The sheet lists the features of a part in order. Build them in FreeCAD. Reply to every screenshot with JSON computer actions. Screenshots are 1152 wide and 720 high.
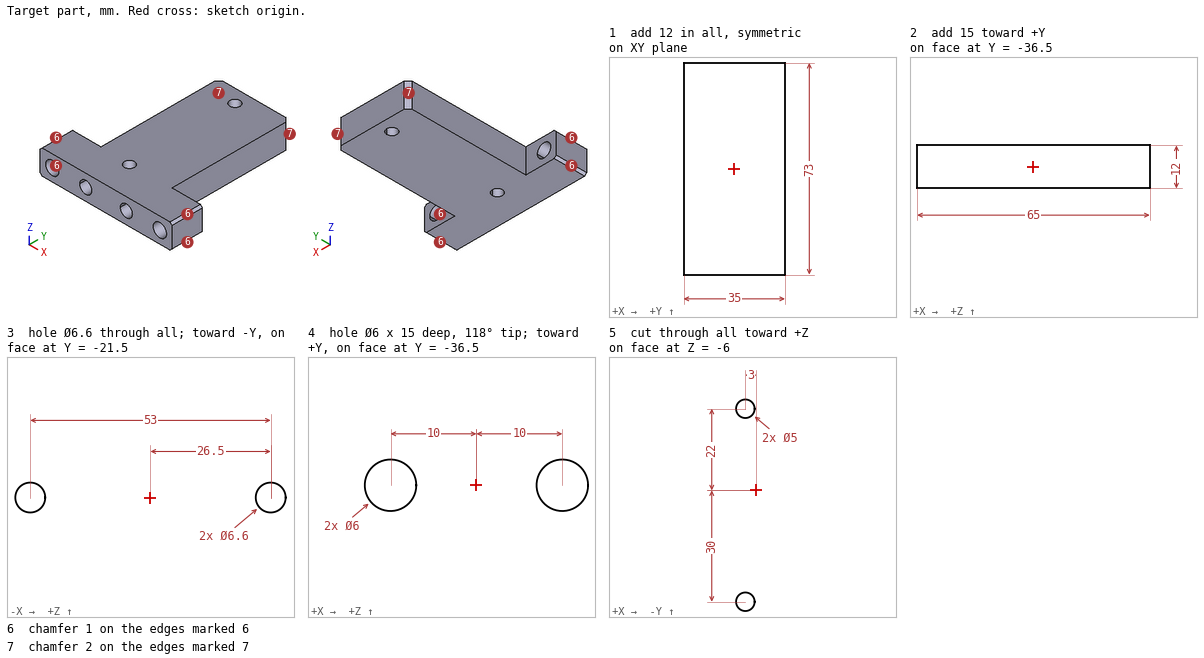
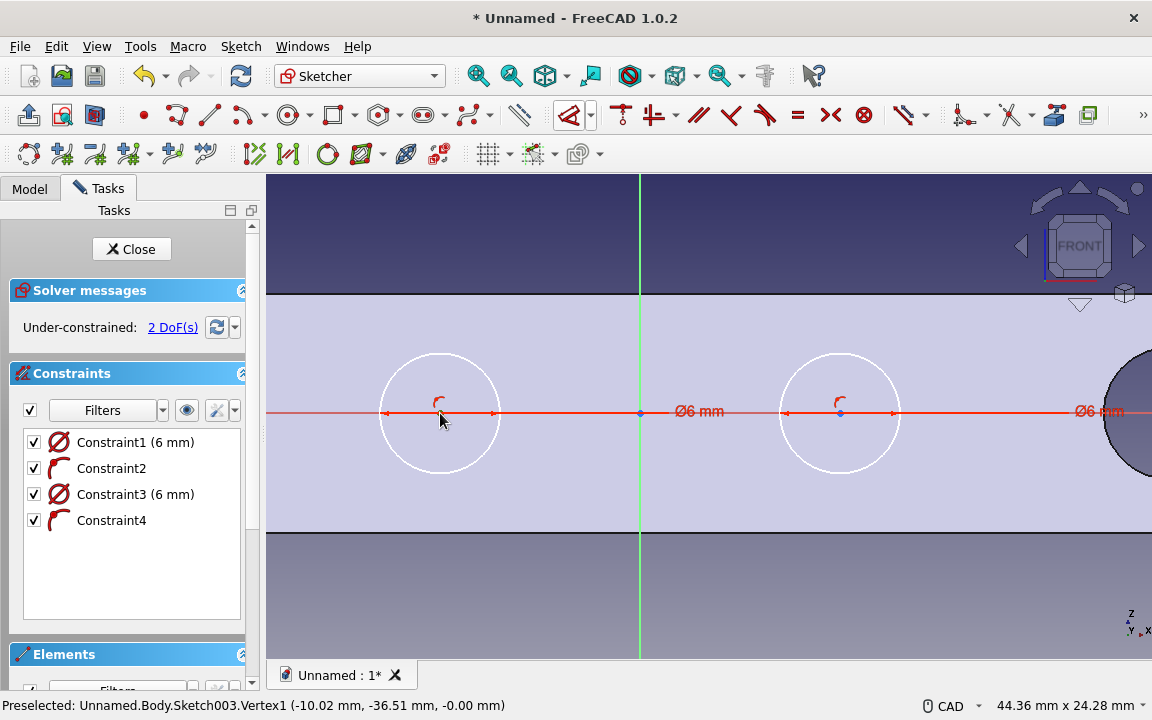
{"action": "key", "text": "l"}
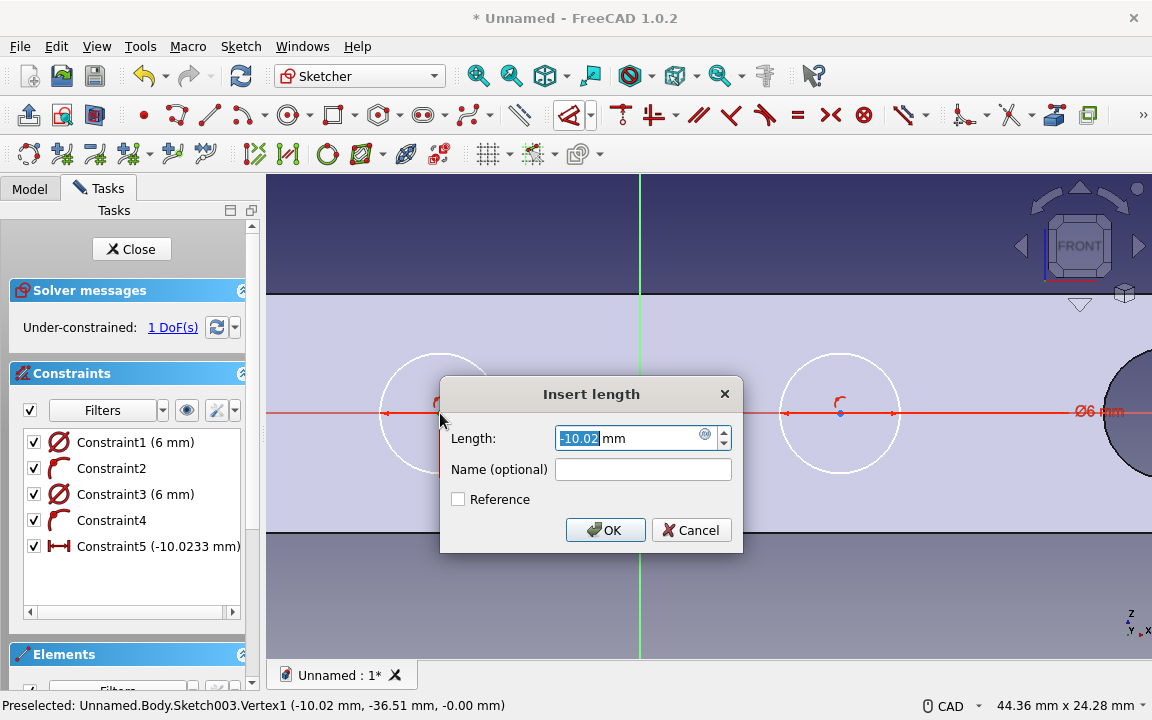
{"action": "type", "text": "-10"}
{"action": "key", "text": "Return"}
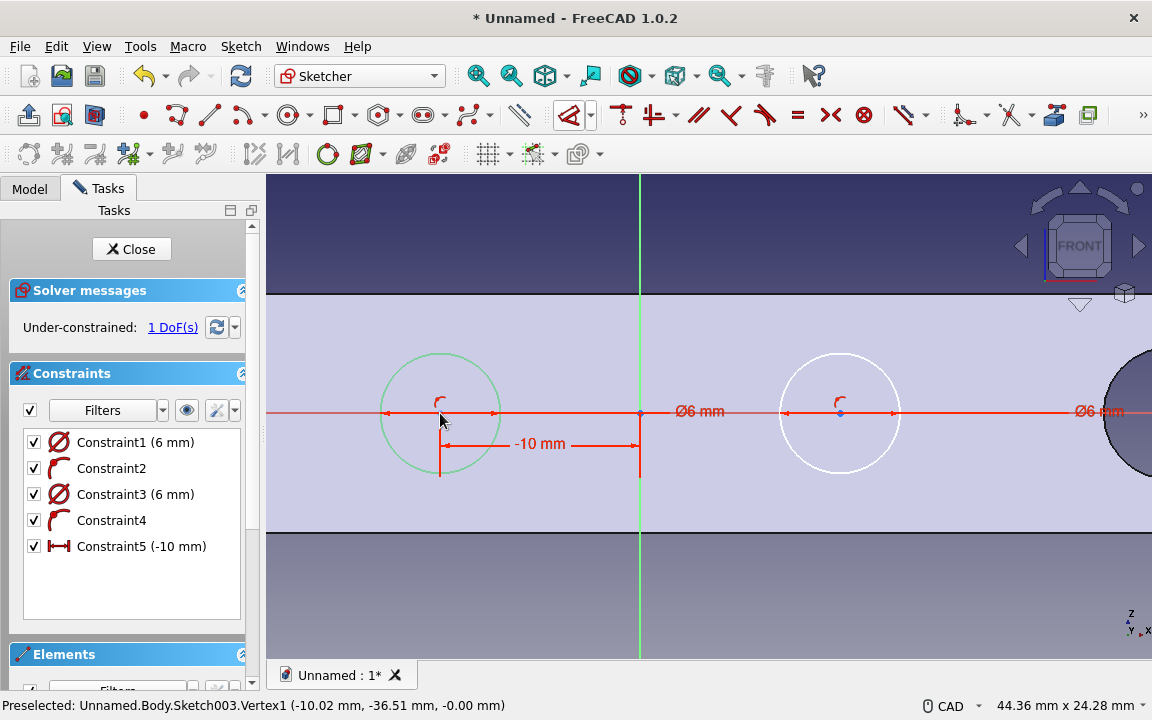
{"action": "left_click", "coordinate": [840, 413]}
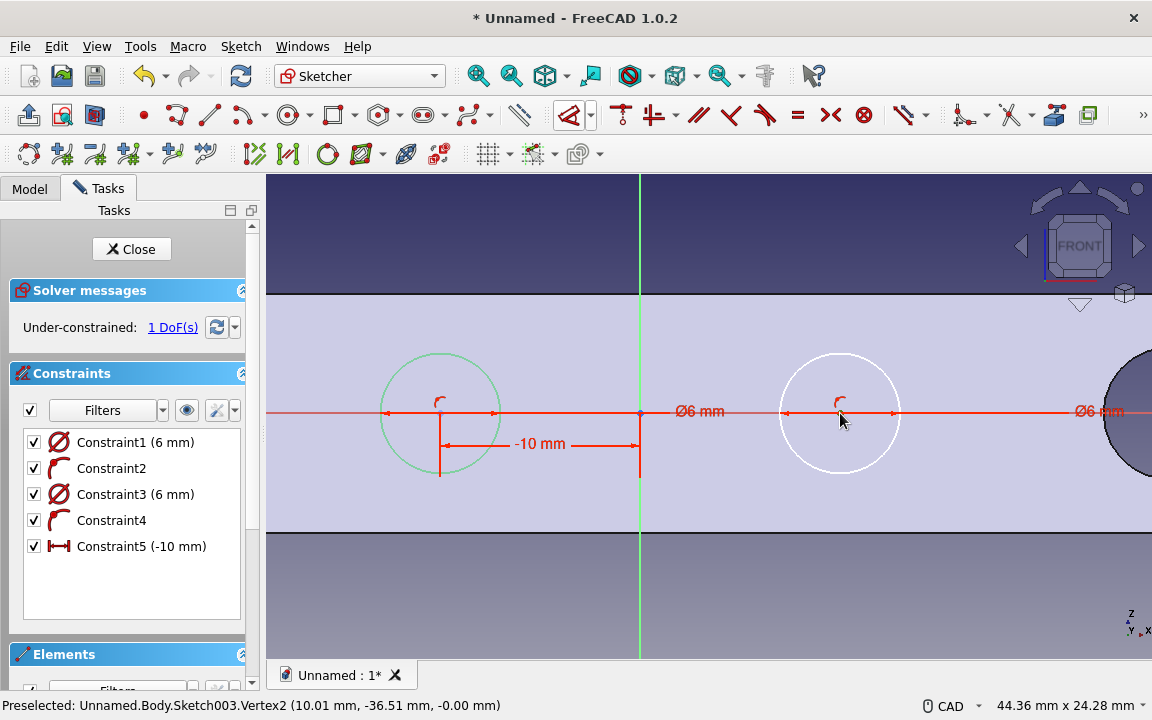
{"action": "left_click", "coordinate": [590, 116]}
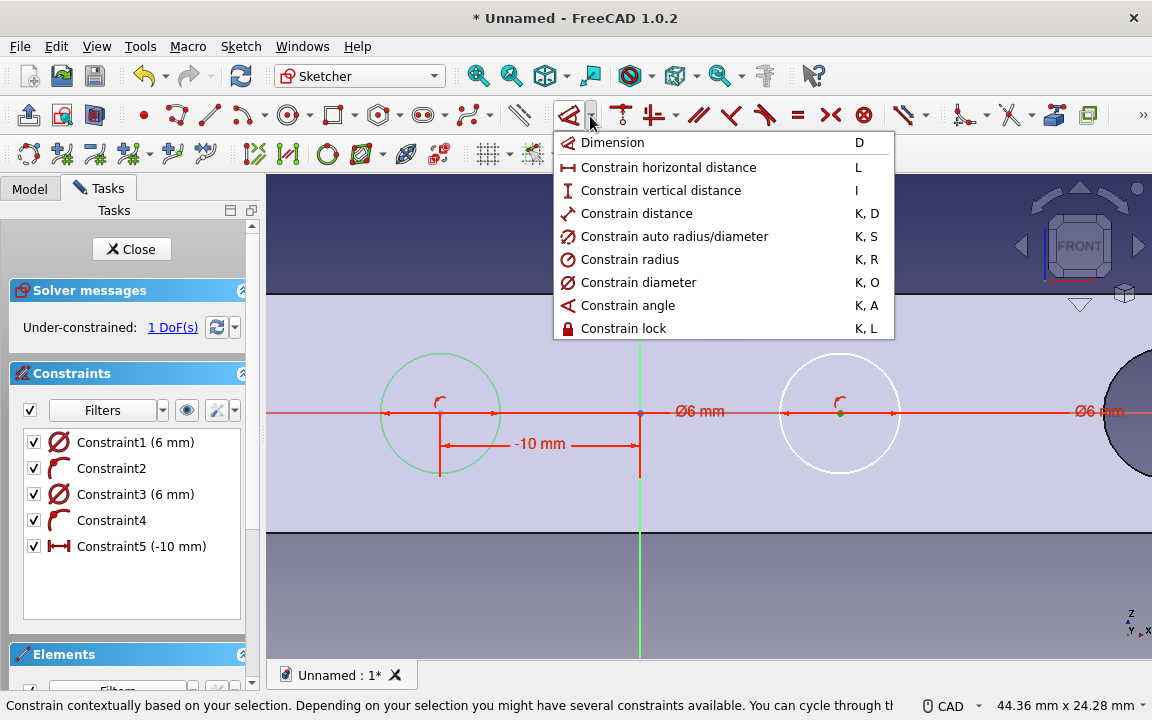
{"action": "left_click", "coordinate": [724, 168]}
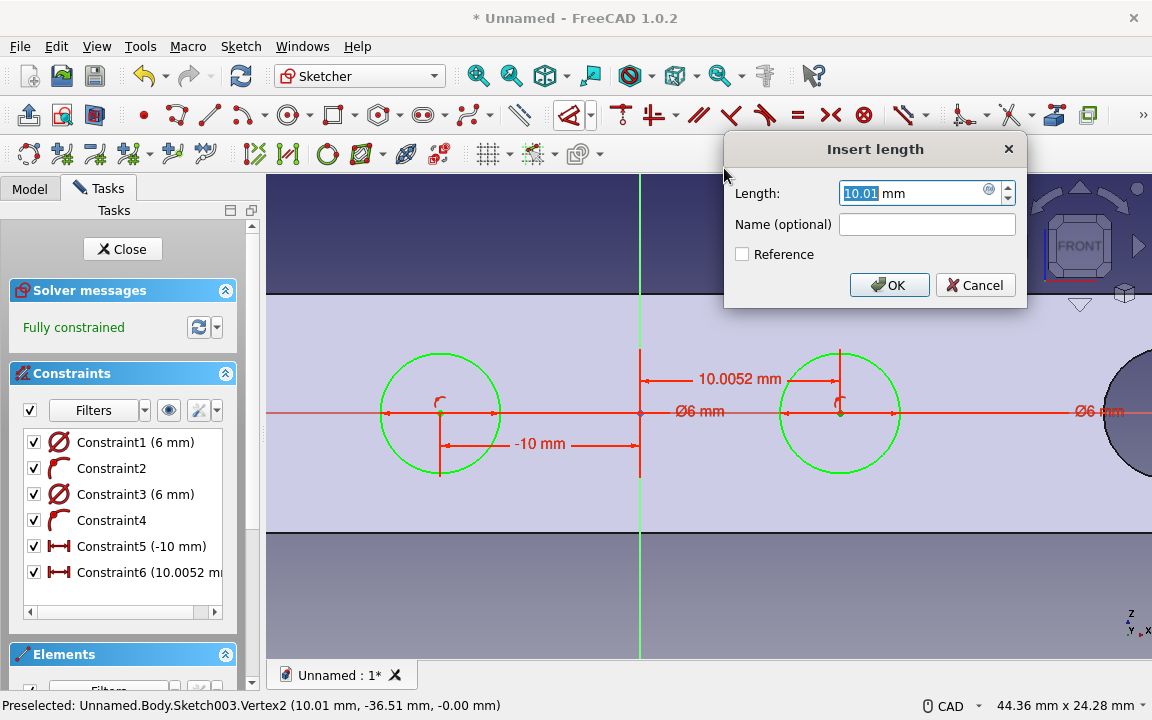
{"action": "type", "text": "10"}
{"action": "key", "text": "Return"}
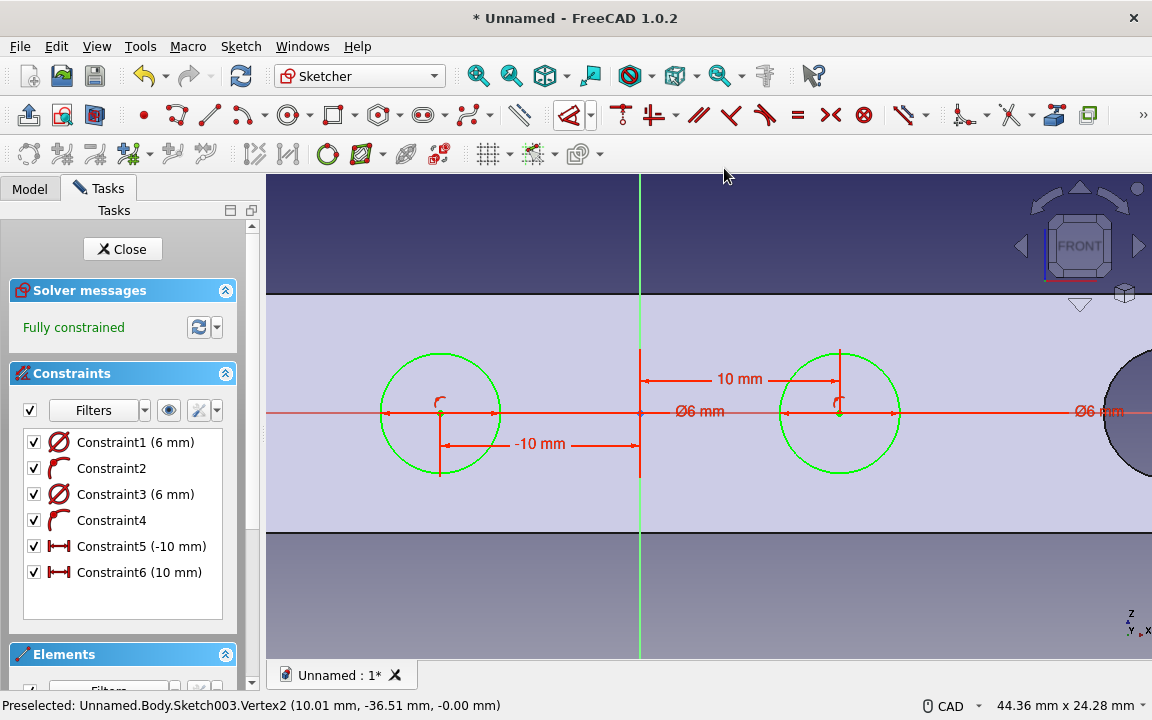
{"action": "left_click", "coordinate": [123, 249]}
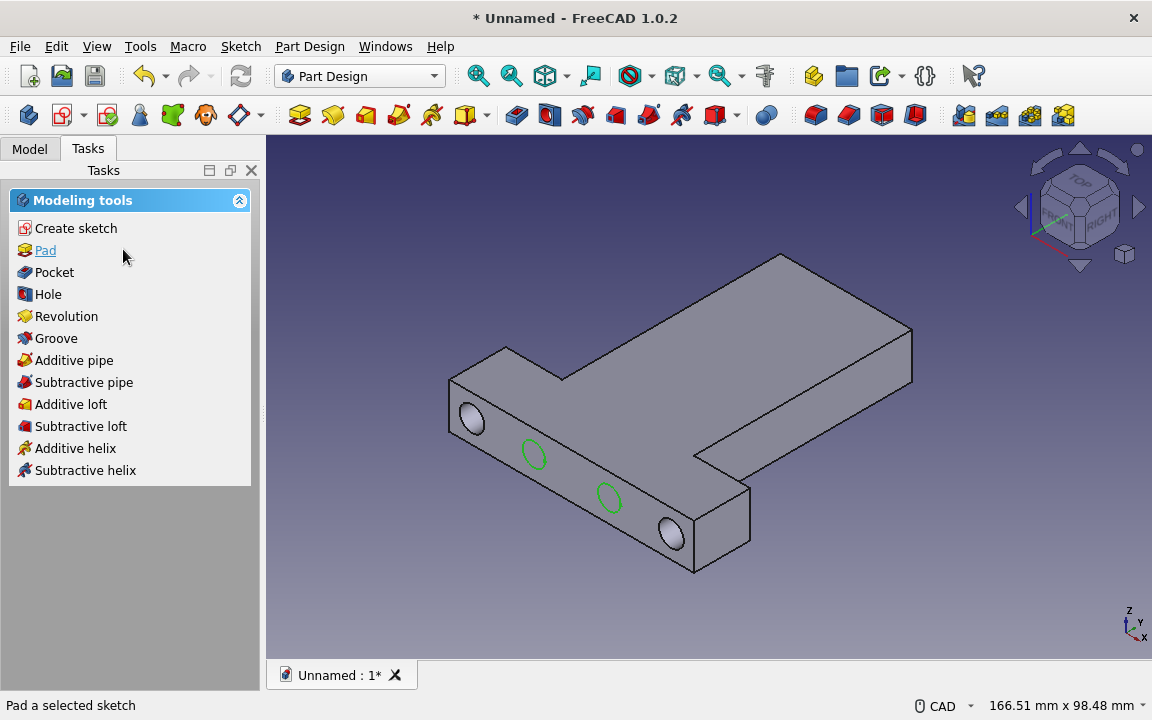
{"action": "left_click", "coordinate": [550, 116]}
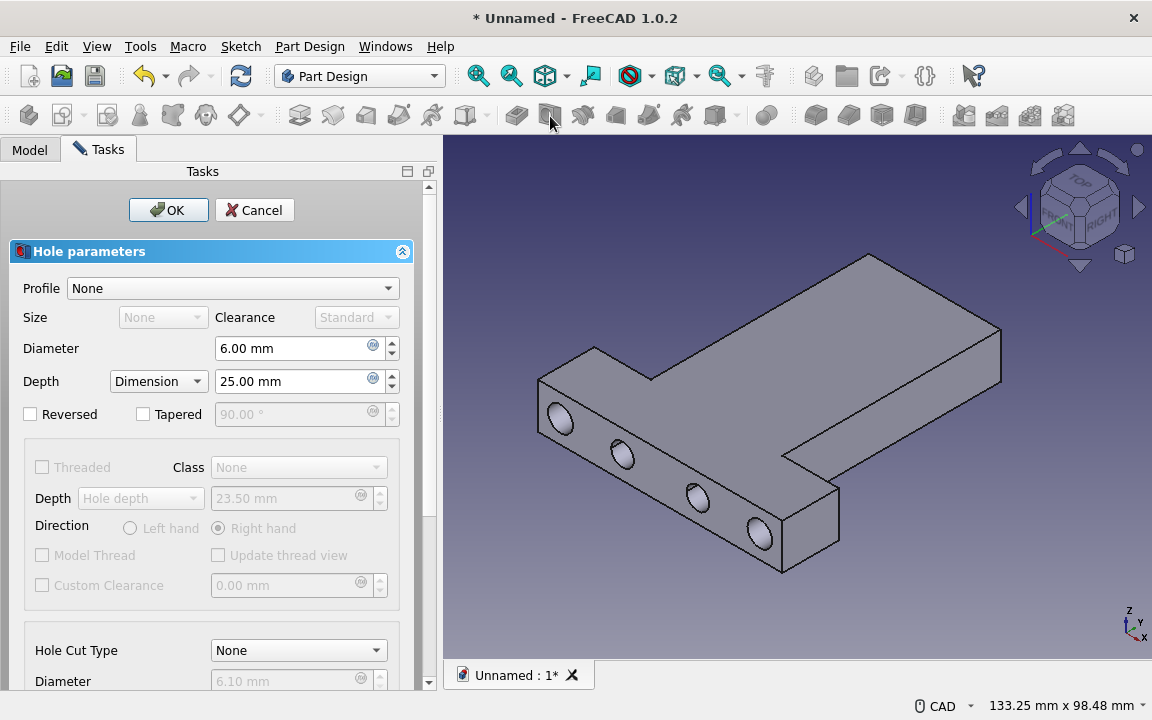
{"action": "triple_click", "coordinate": [300, 348]}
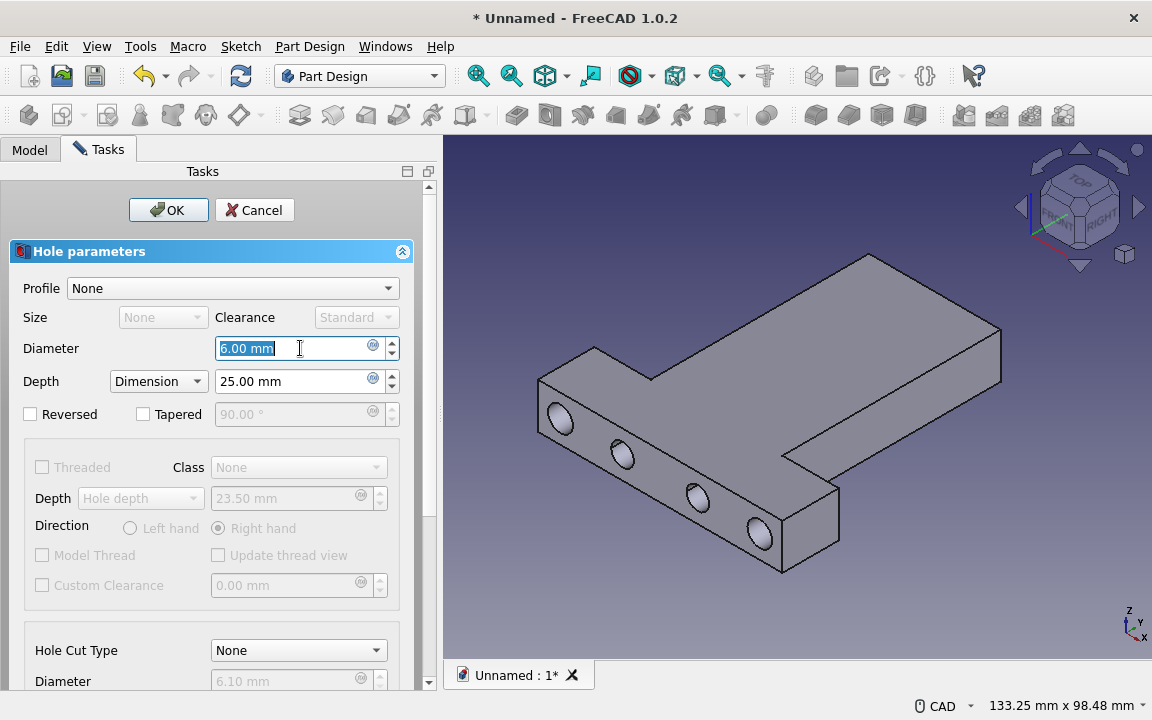
{"action": "type", "text": "6"}
{"action": "key", "text": "Tab"}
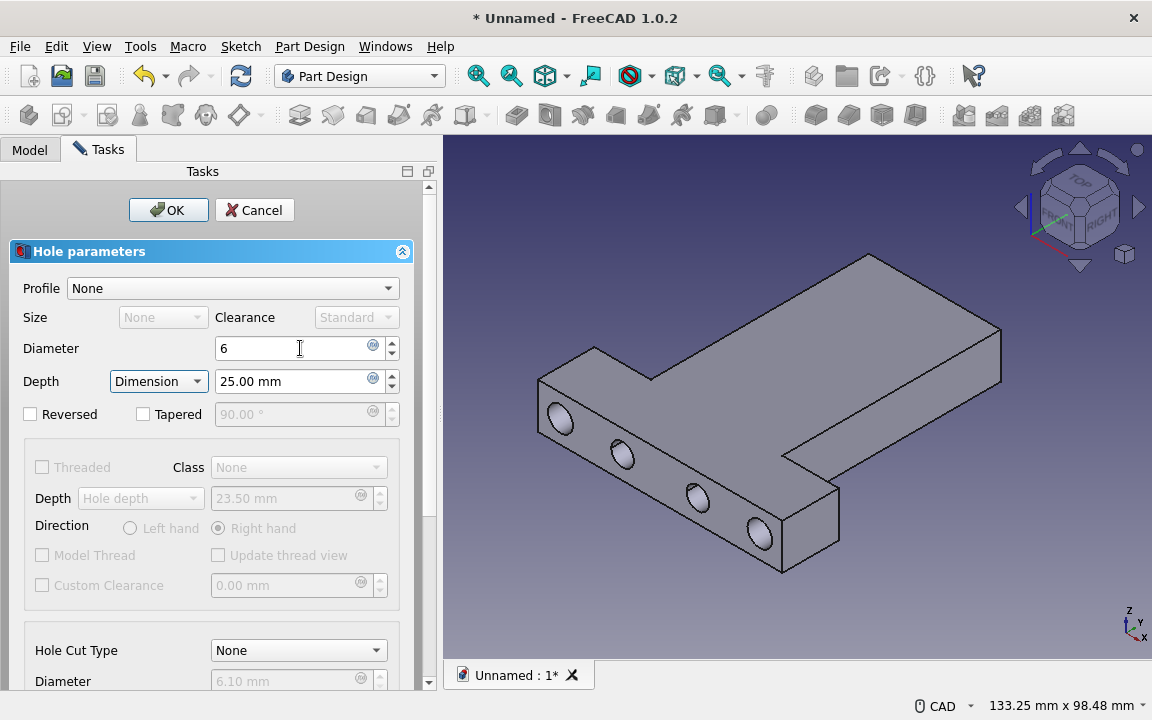
{"action": "triple_click", "coordinate": [300, 382]}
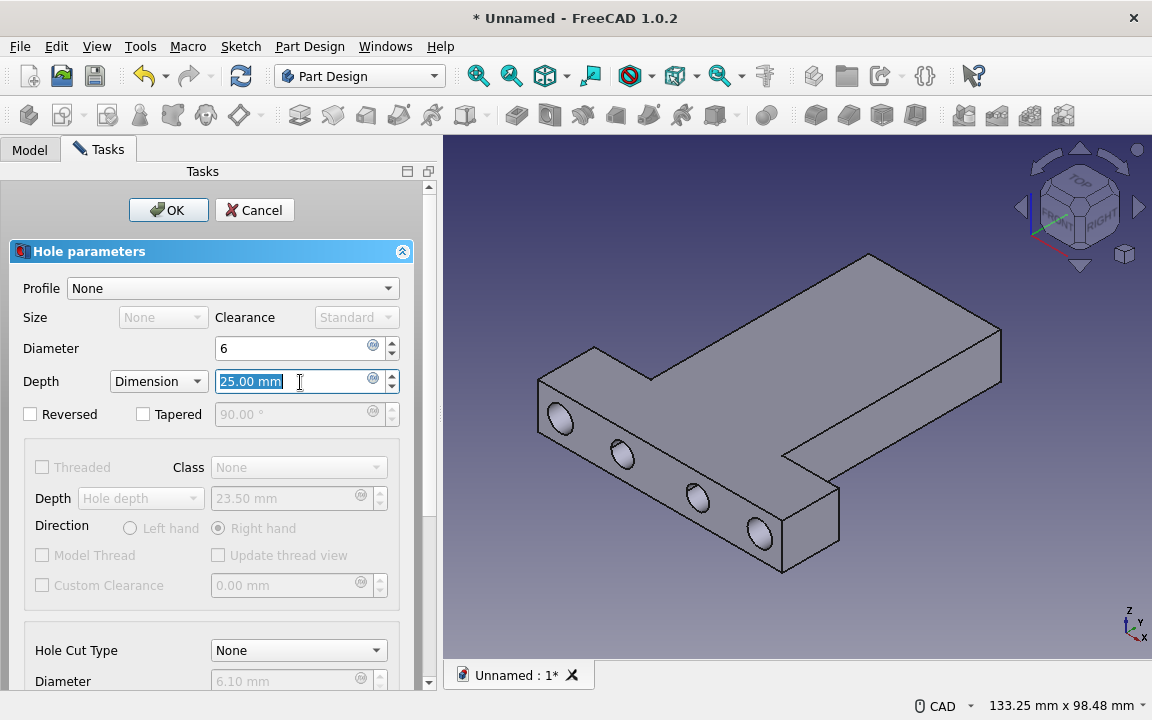
{"action": "type", "text": "15"}
{"action": "key", "text": "Tab"}